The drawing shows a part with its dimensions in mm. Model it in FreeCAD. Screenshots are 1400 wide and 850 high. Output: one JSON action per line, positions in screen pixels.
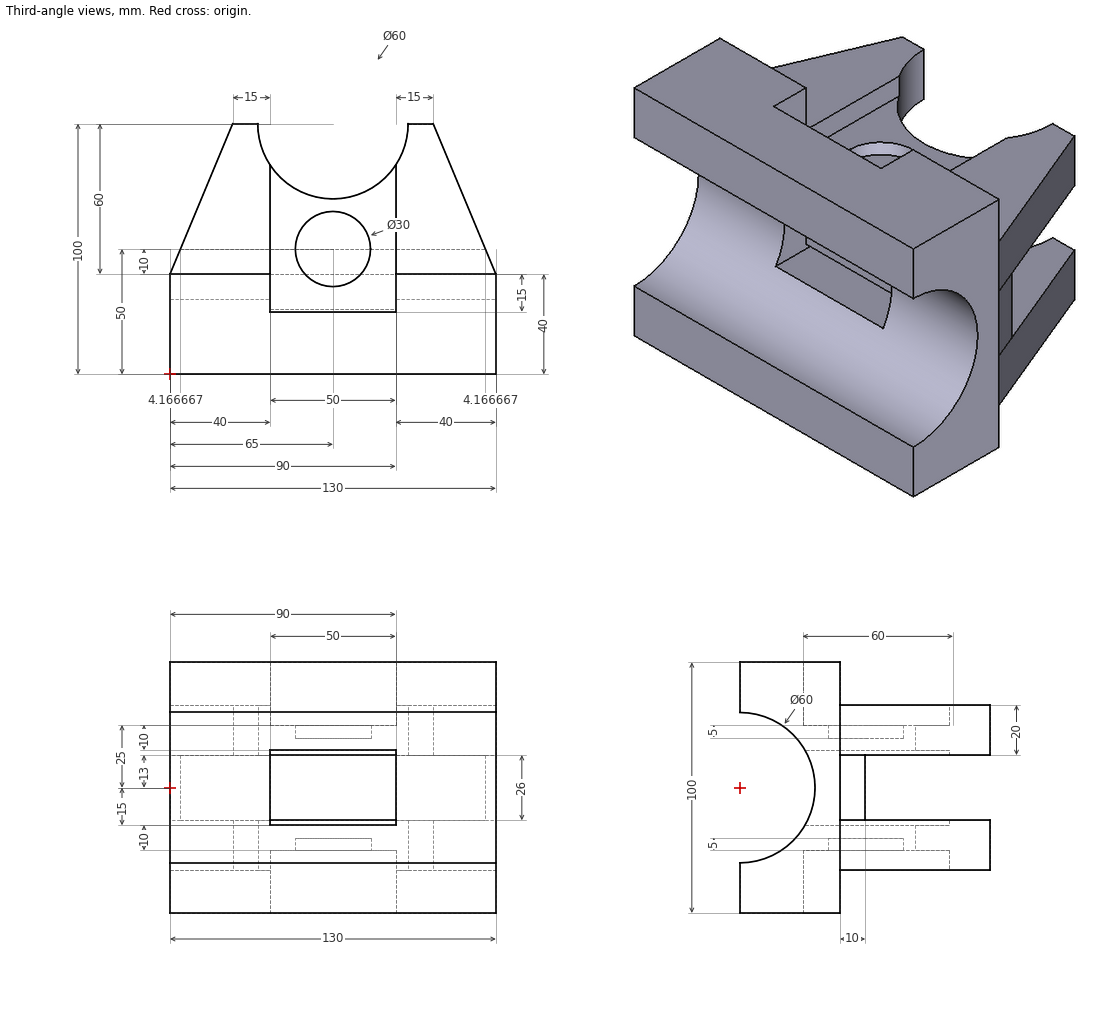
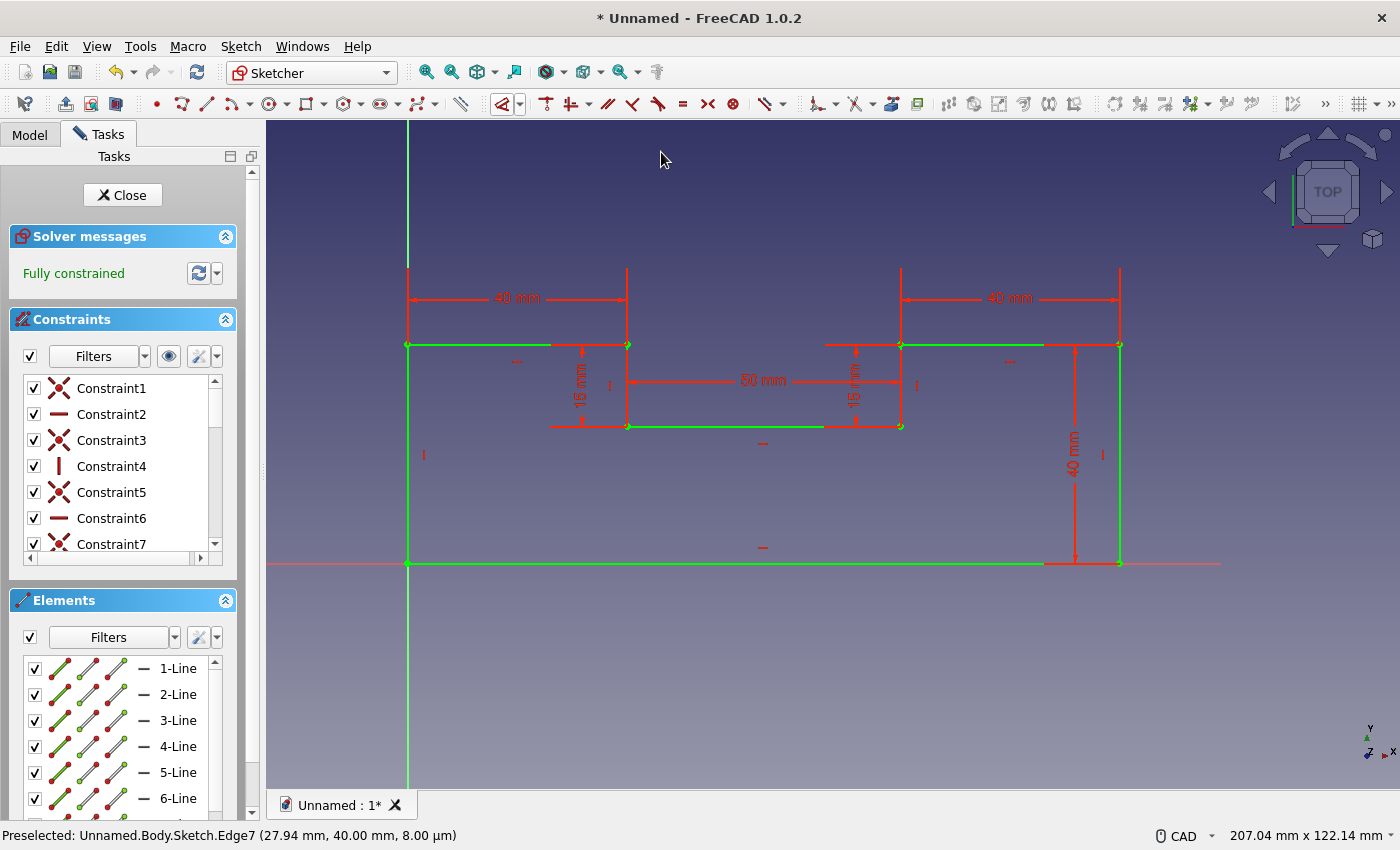
{"action": "left_click", "coordinate": [123, 195]}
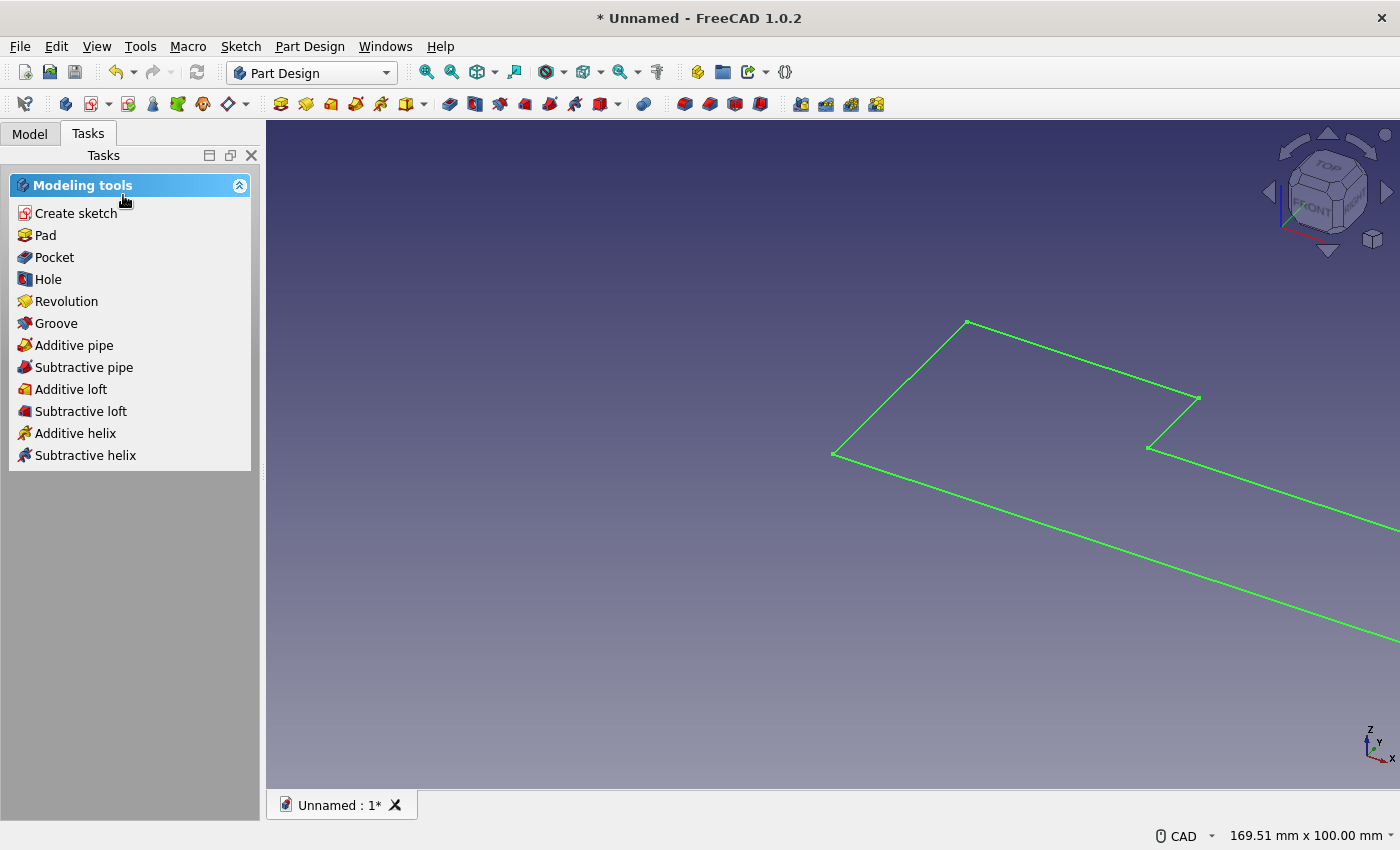
{"action": "left_click", "coordinate": [281, 104]}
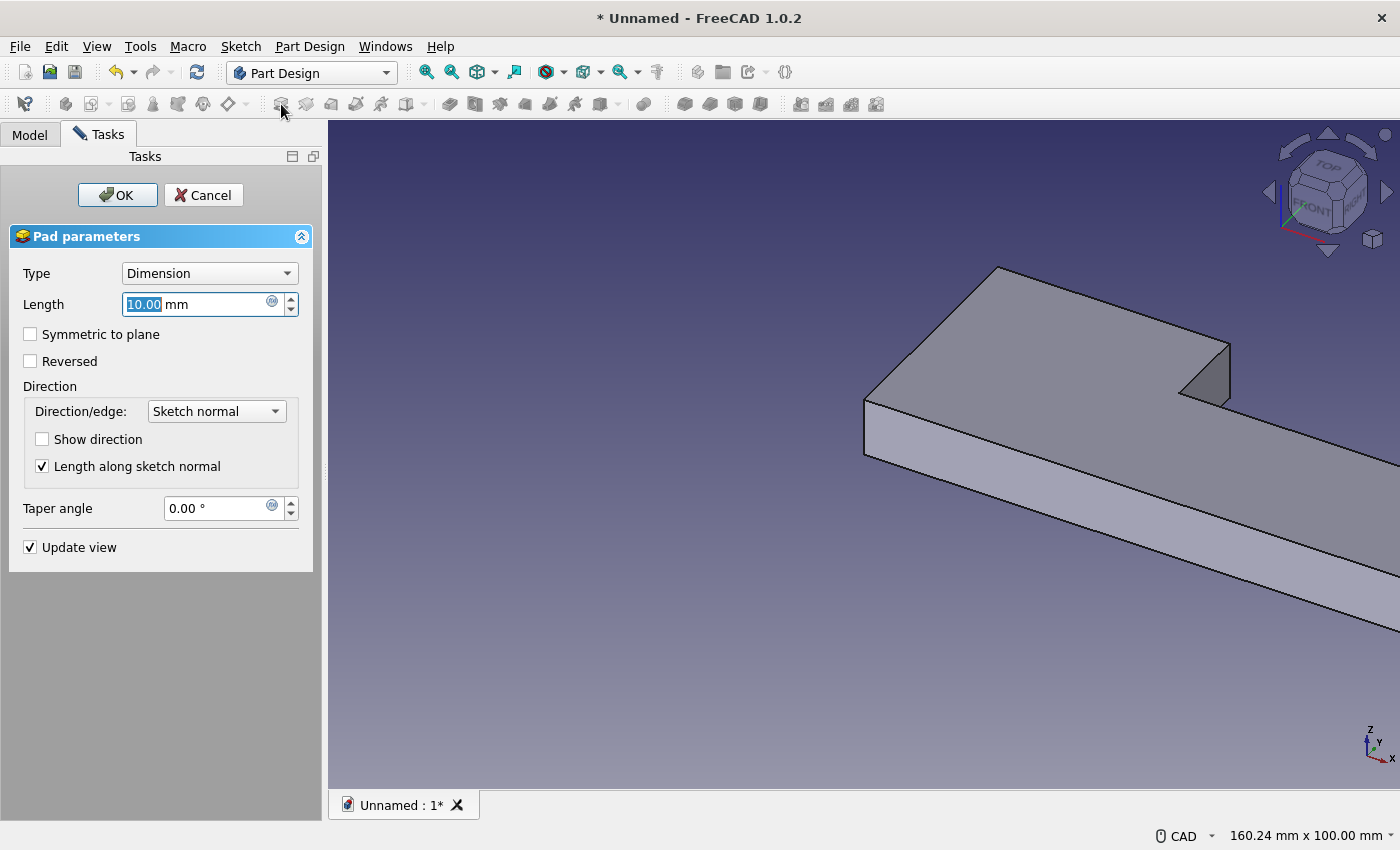
{"action": "type", "text": "100"}
{"action": "key", "text": "Tab"}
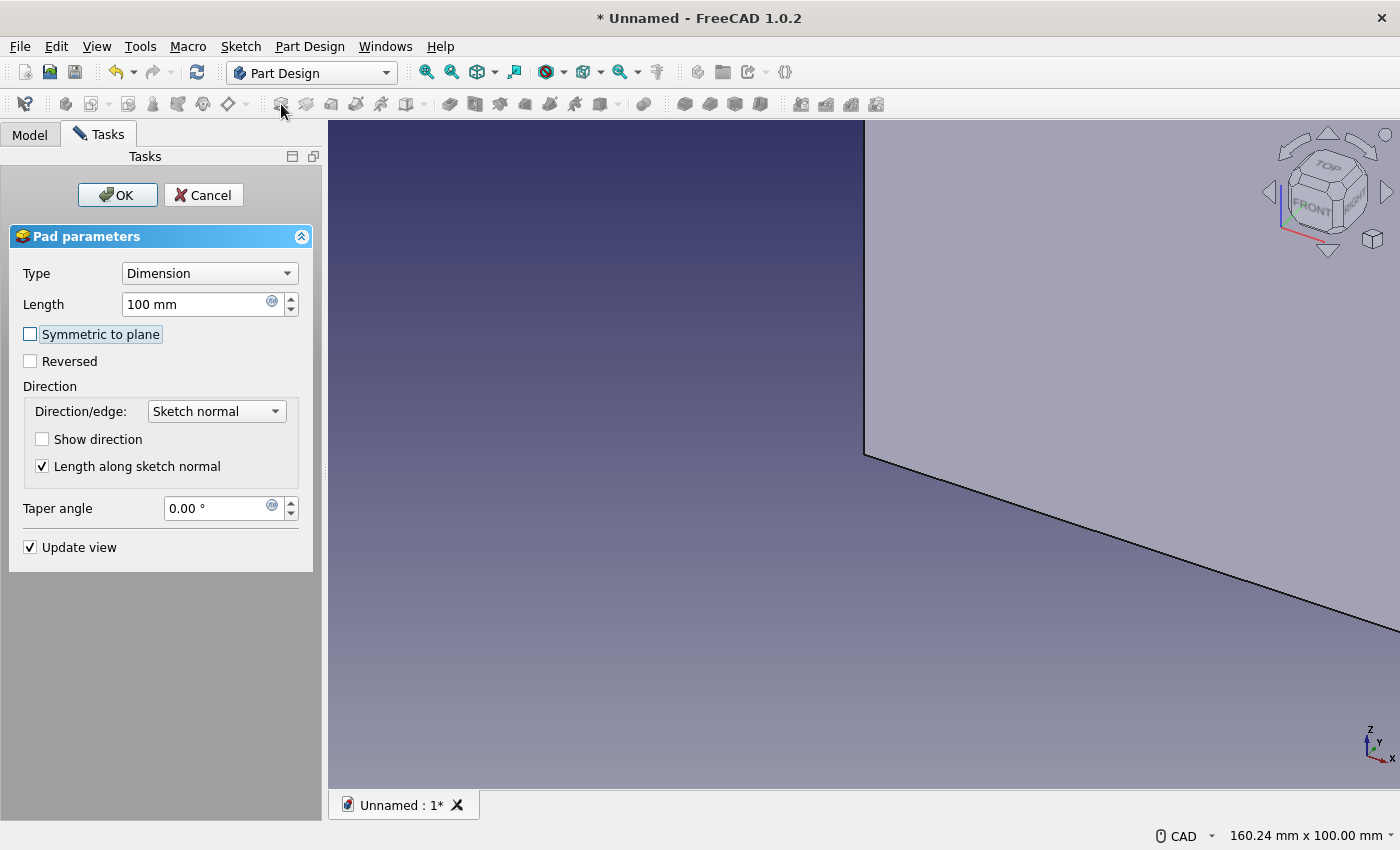
{"action": "left_click", "coordinate": [31, 334]}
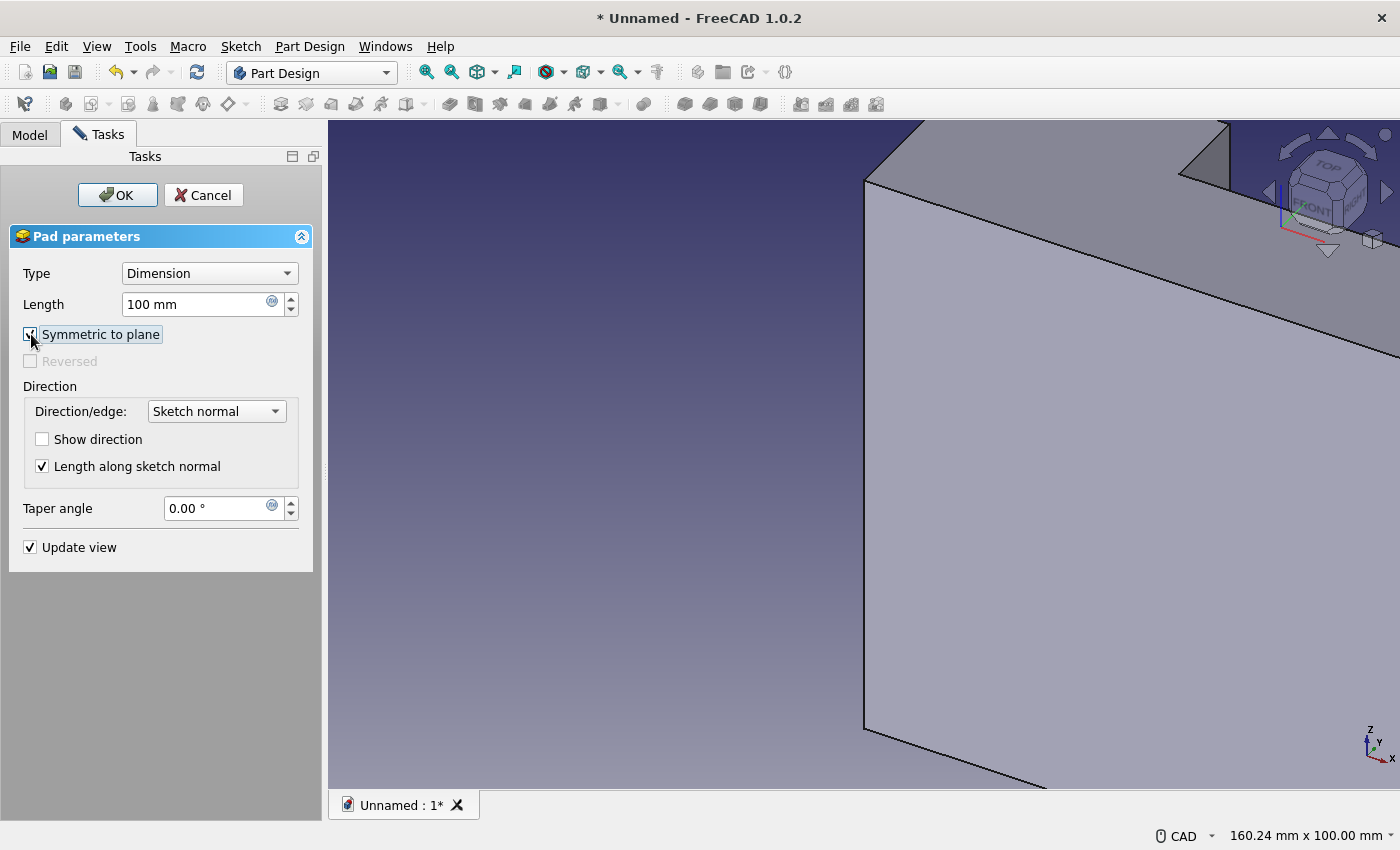
{"action": "left_click", "coordinate": [118, 195]}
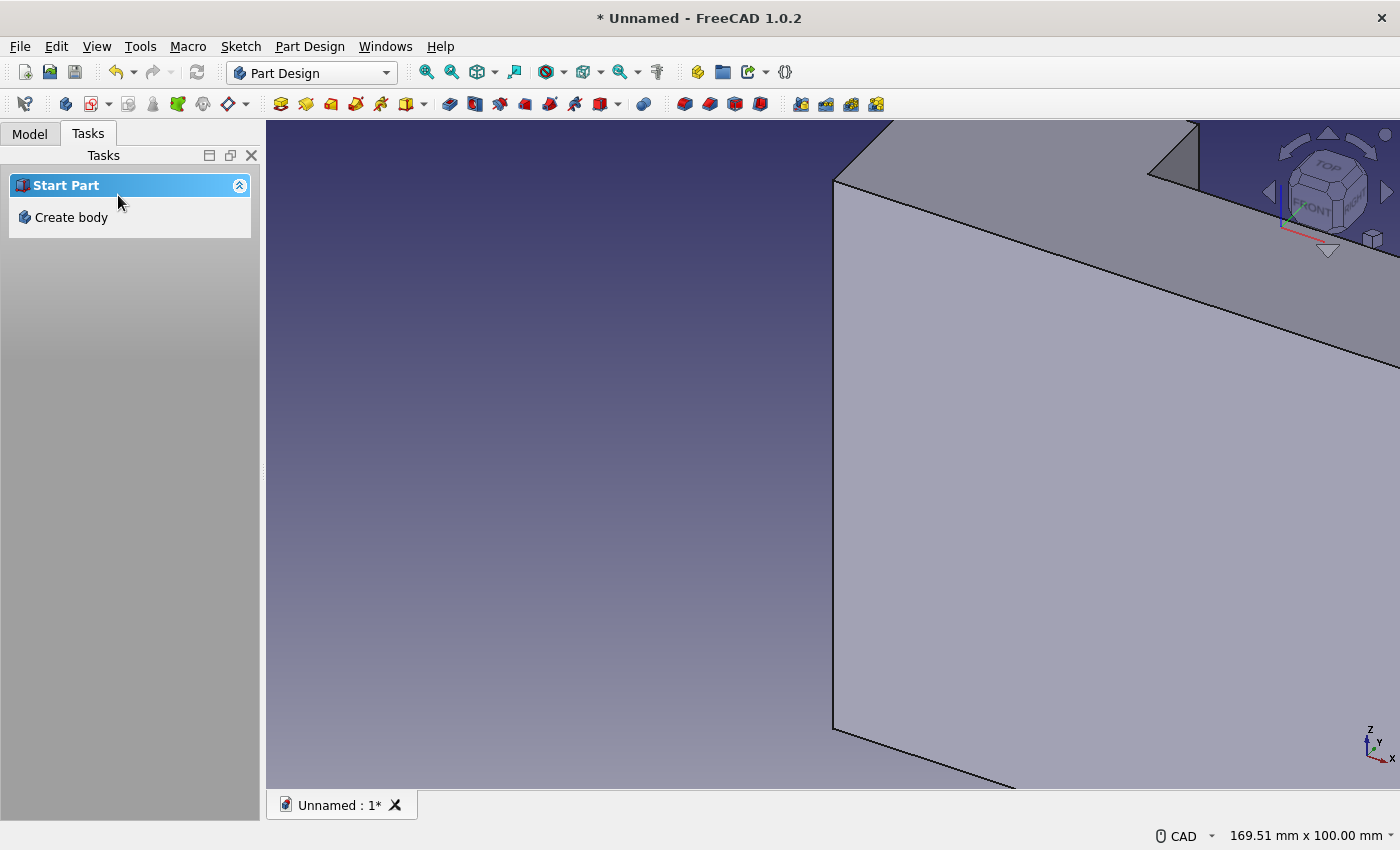
{"action": "left_click", "coordinate": [427, 72]}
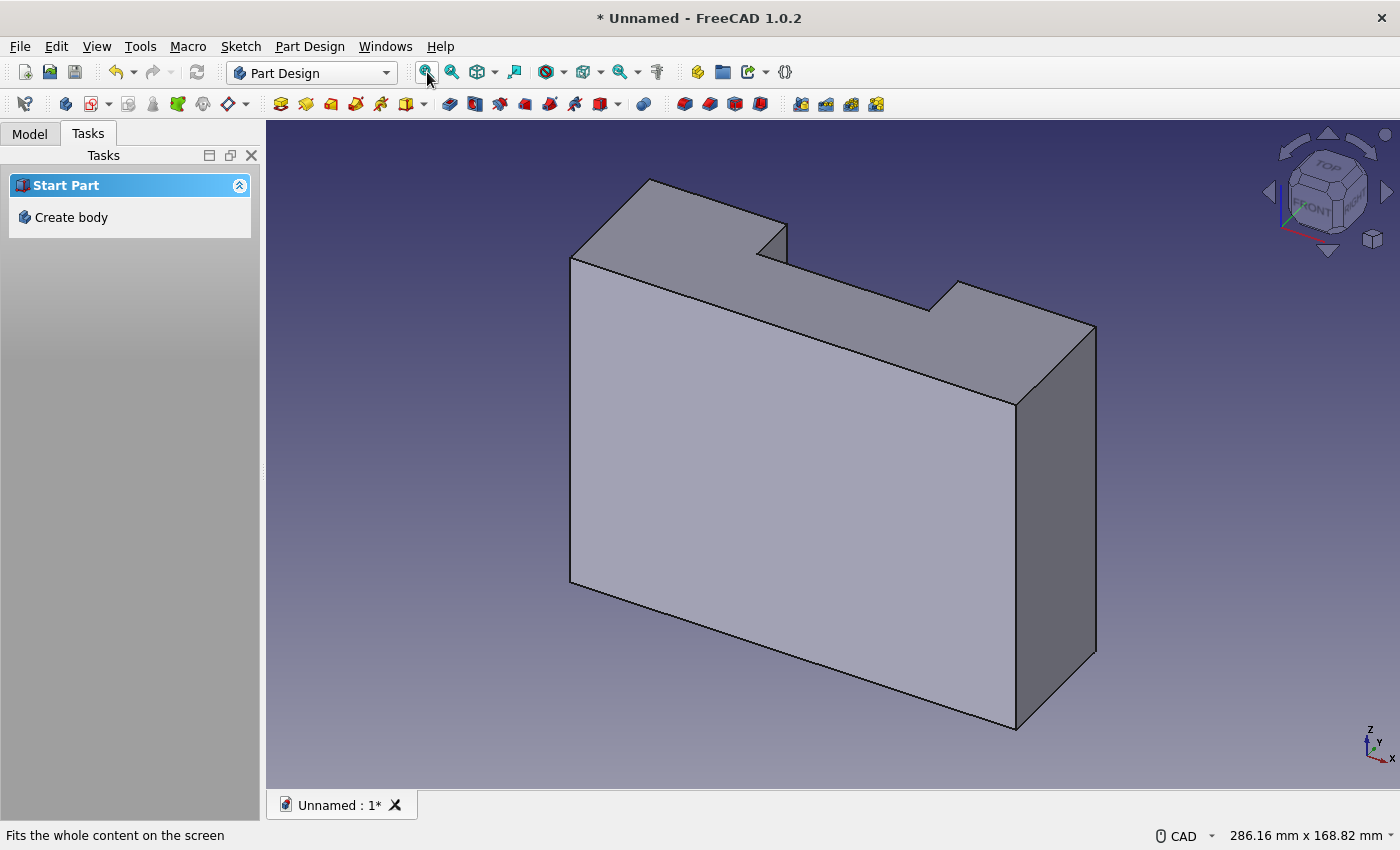
{"action": "left_click", "coordinate": [1056, 435]}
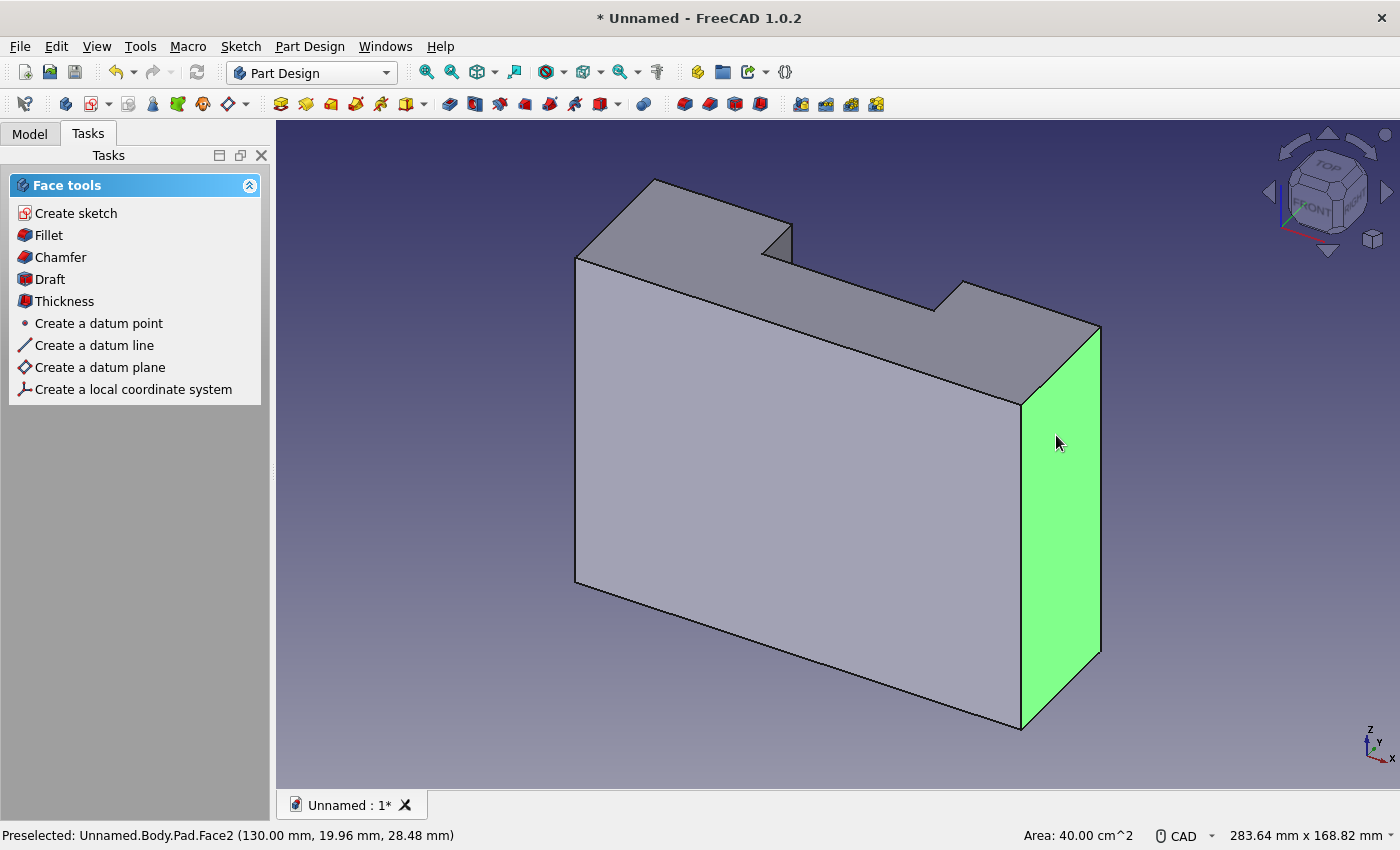
{"action": "left_click", "coordinate": [90, 104]}